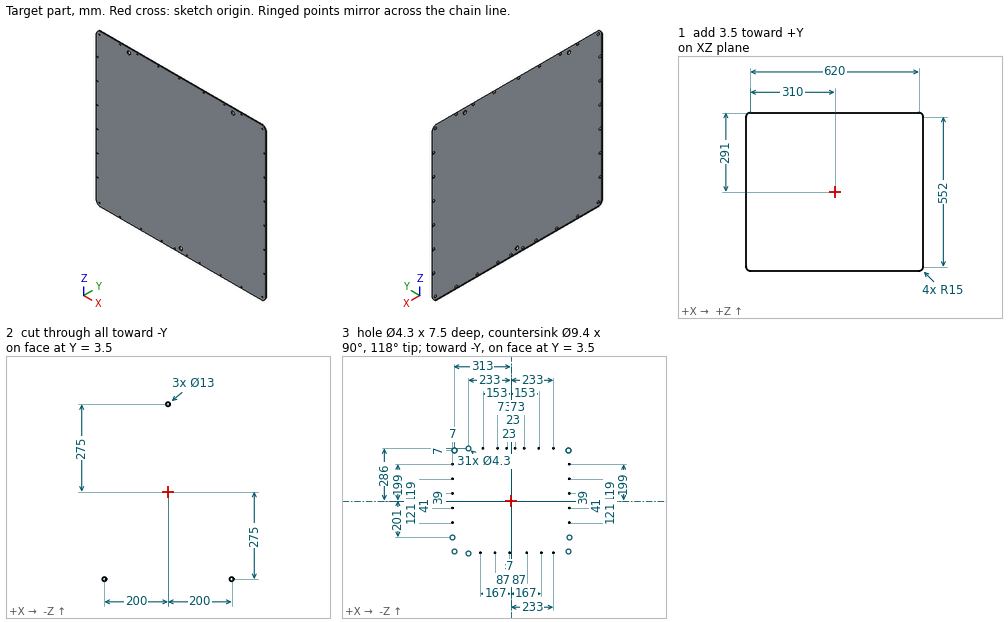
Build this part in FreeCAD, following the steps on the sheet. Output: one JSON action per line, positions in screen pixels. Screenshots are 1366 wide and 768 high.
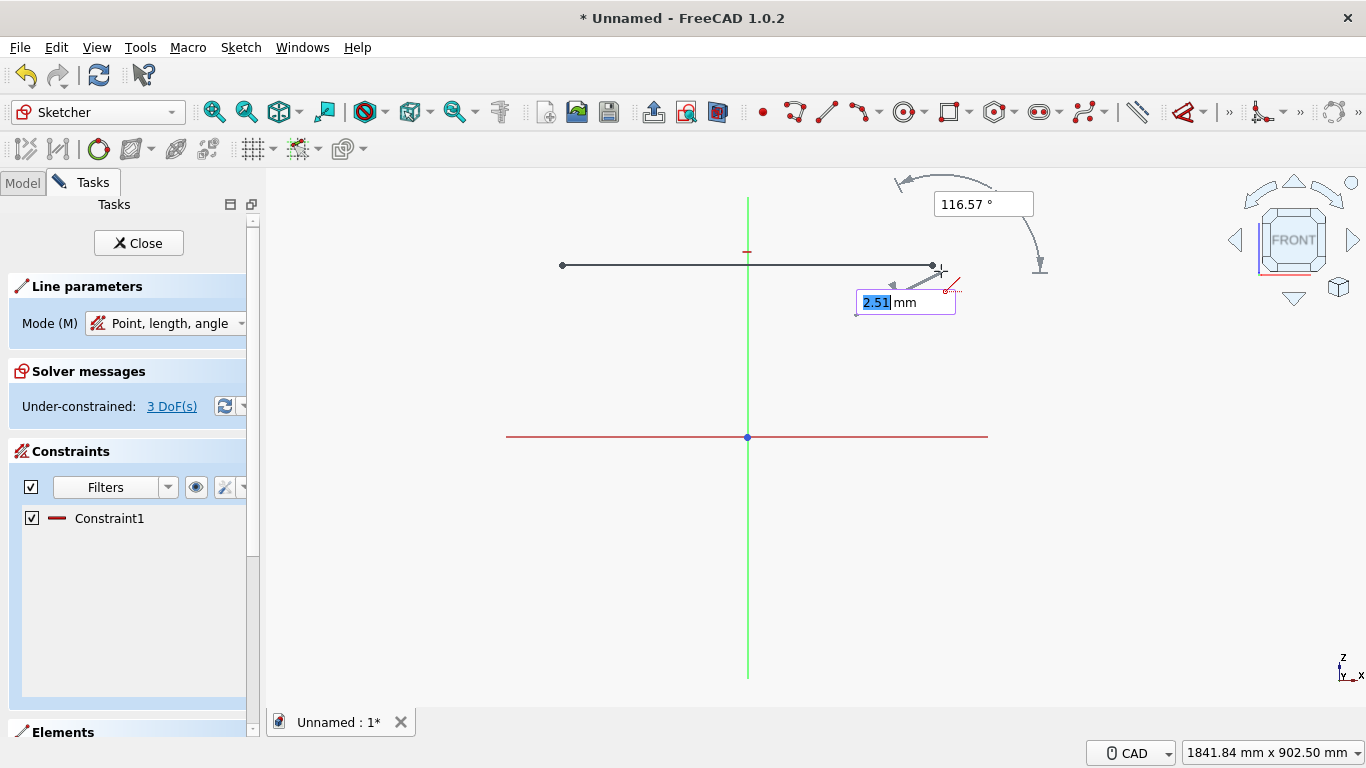
{"action": "left_click", "coordinate": [942, 602]}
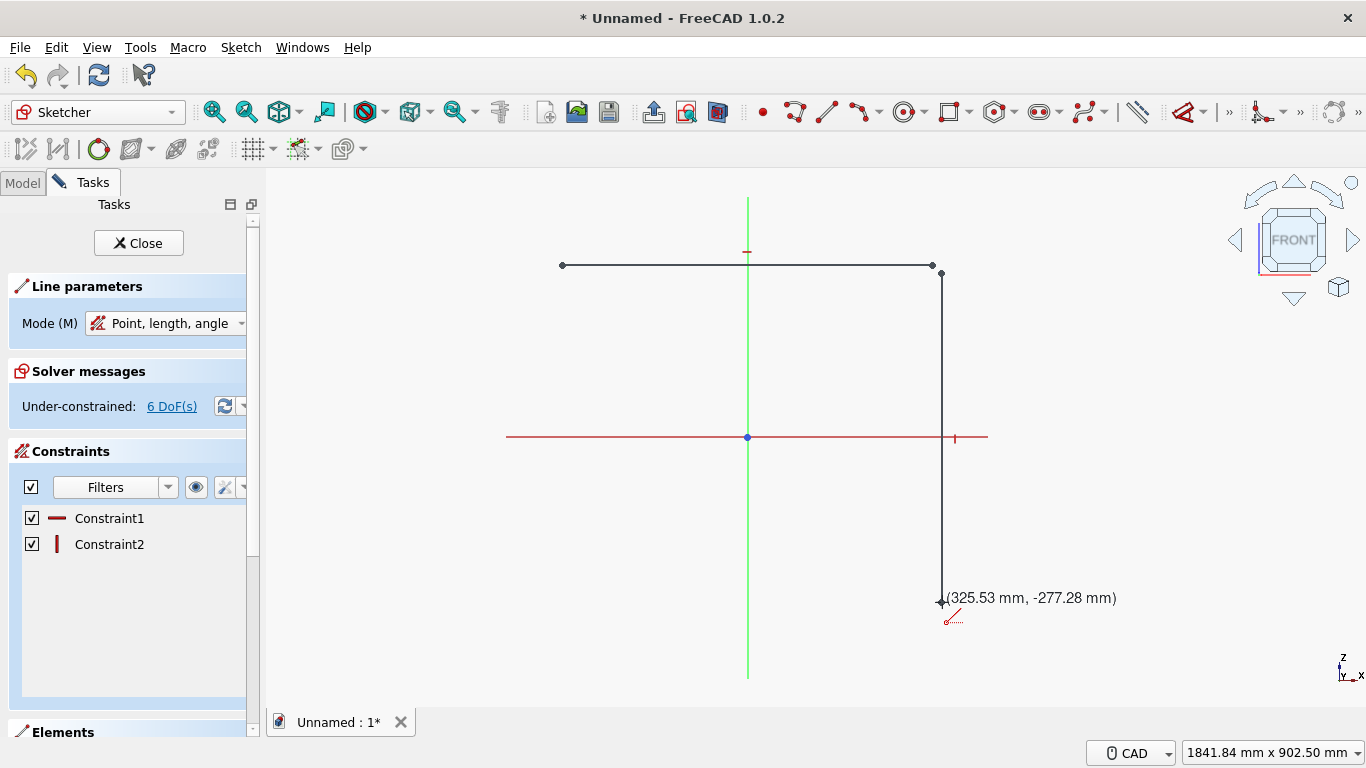
{"action": "scroll", "coordinate": [933, 611], "scroll_direction": "up", "scroll_amount": 2}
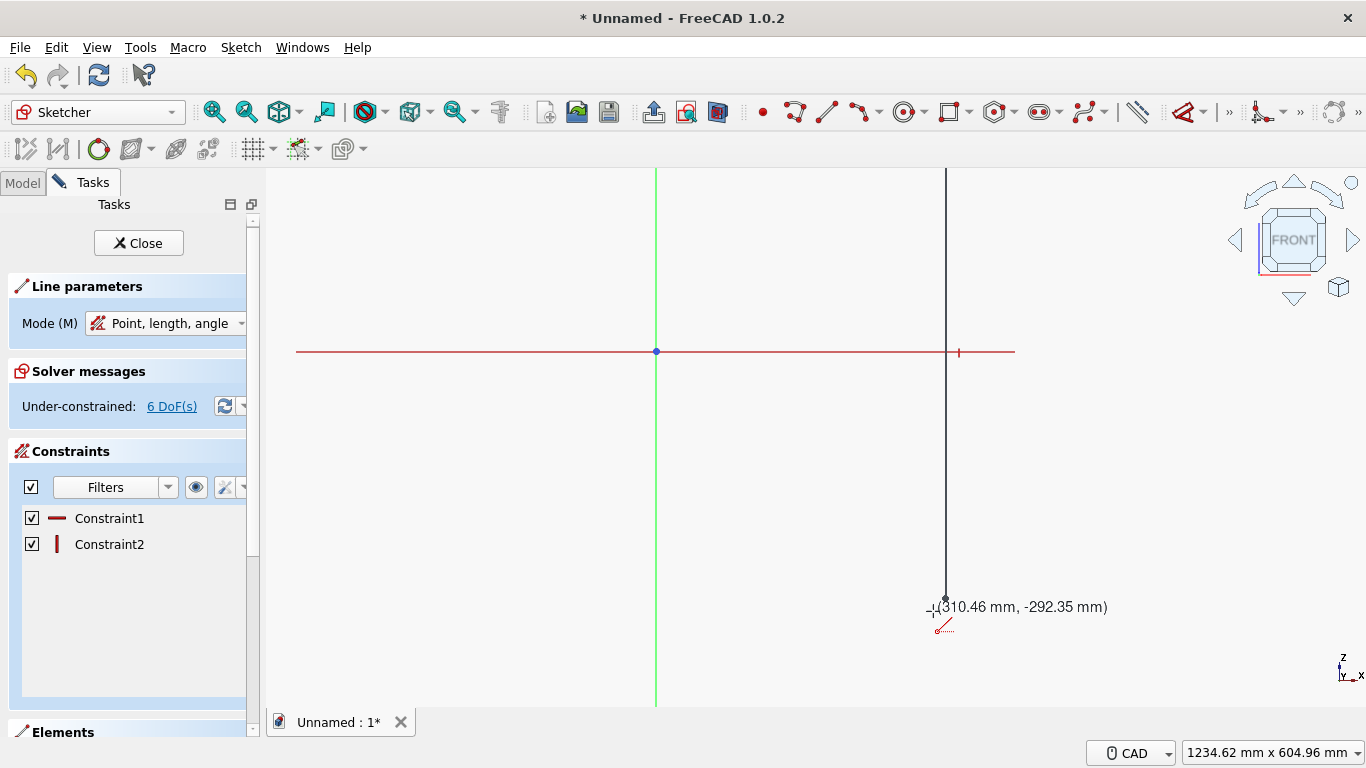
{"action": "left_click", "coordinate": [932, 611]}
{"action": "left_click", "coordinate": [380, 611]}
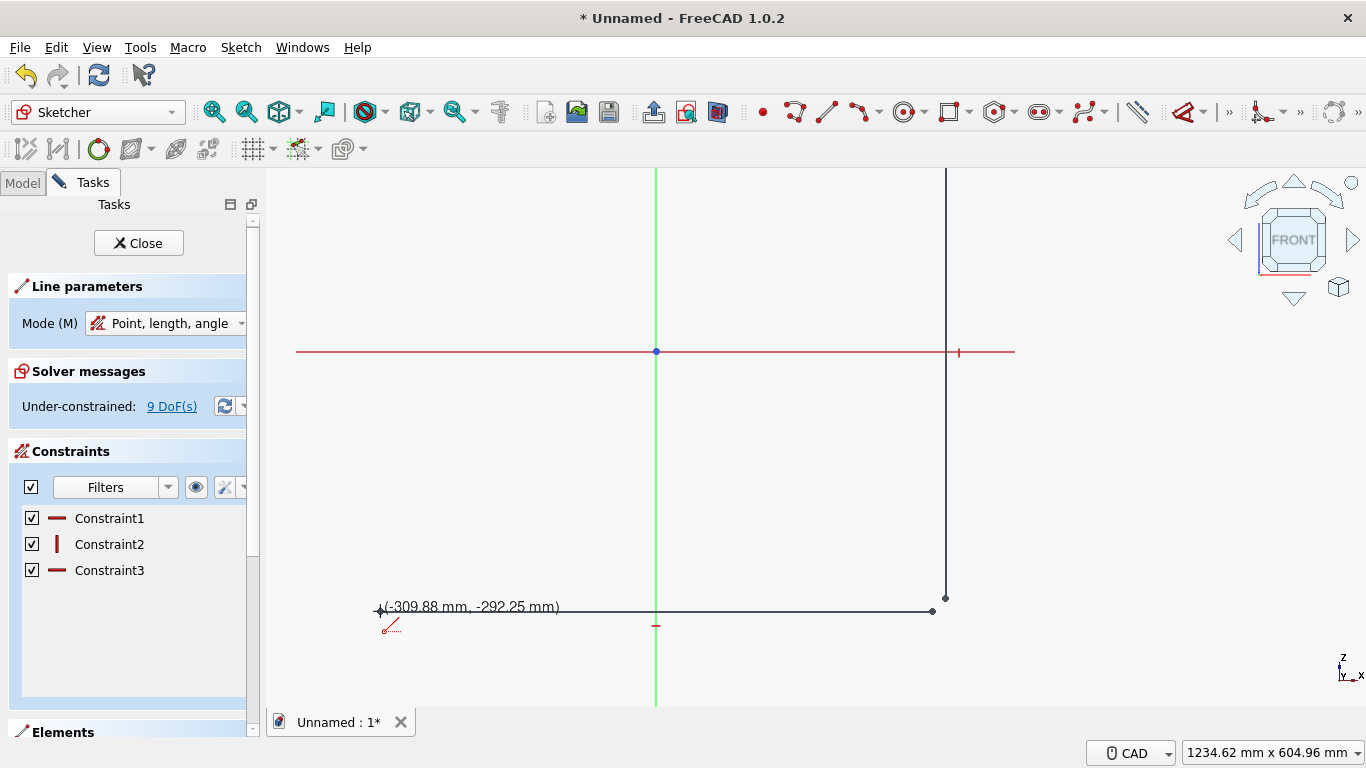
{"action": "left_click", "coordinate": [367, 598]}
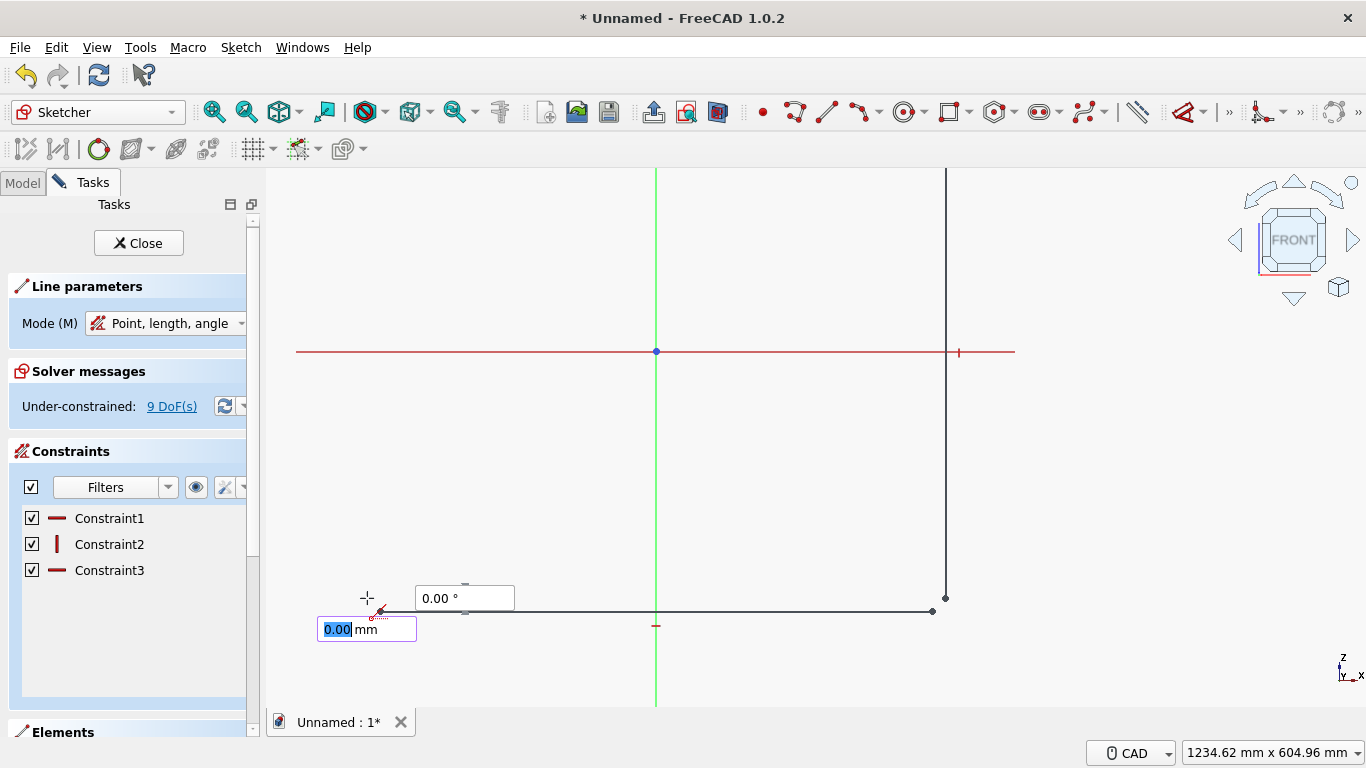
{"action": "scroll", "coordinate": [933, 612], "scroll_direction": "down", "scroll_amount": 2}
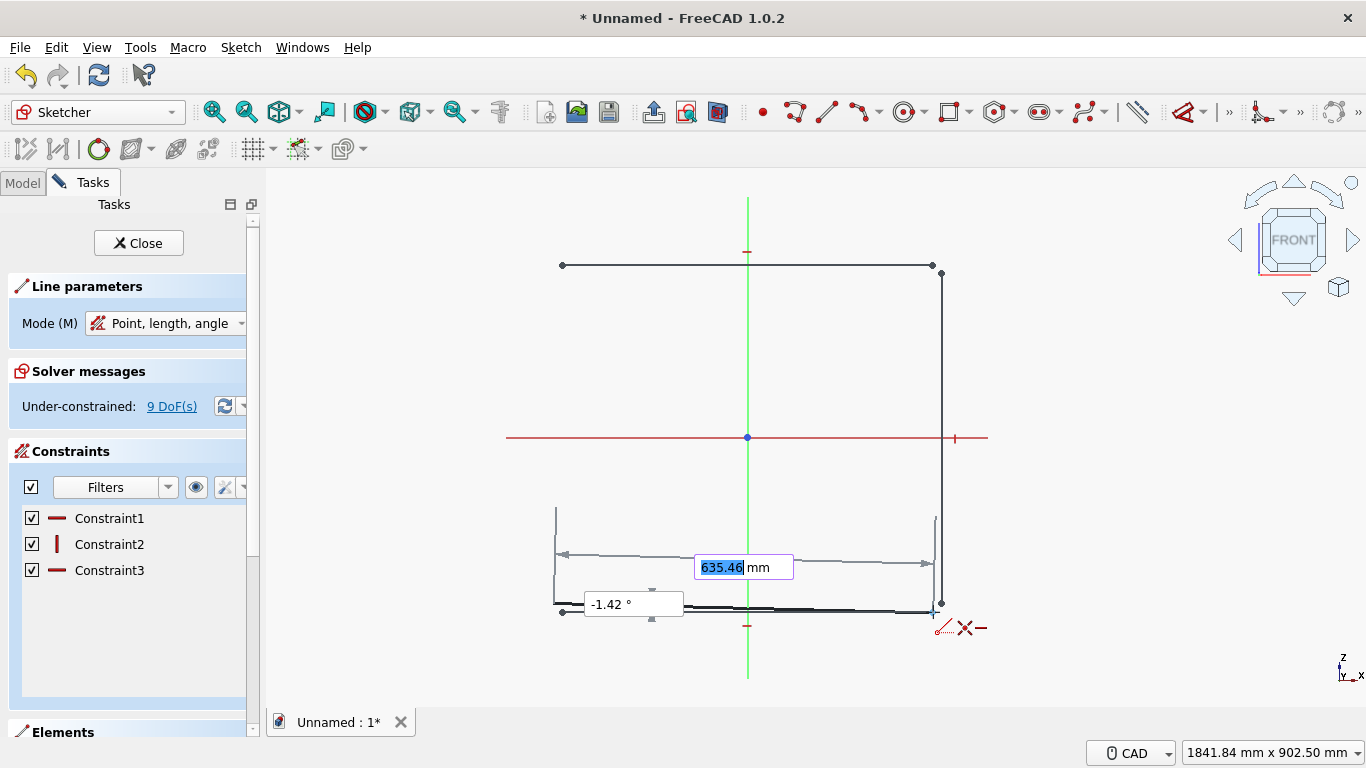
{"action": "scroll", "coordinate": [553, 273], "scroll_direction": "up", "scroll_amount": 2}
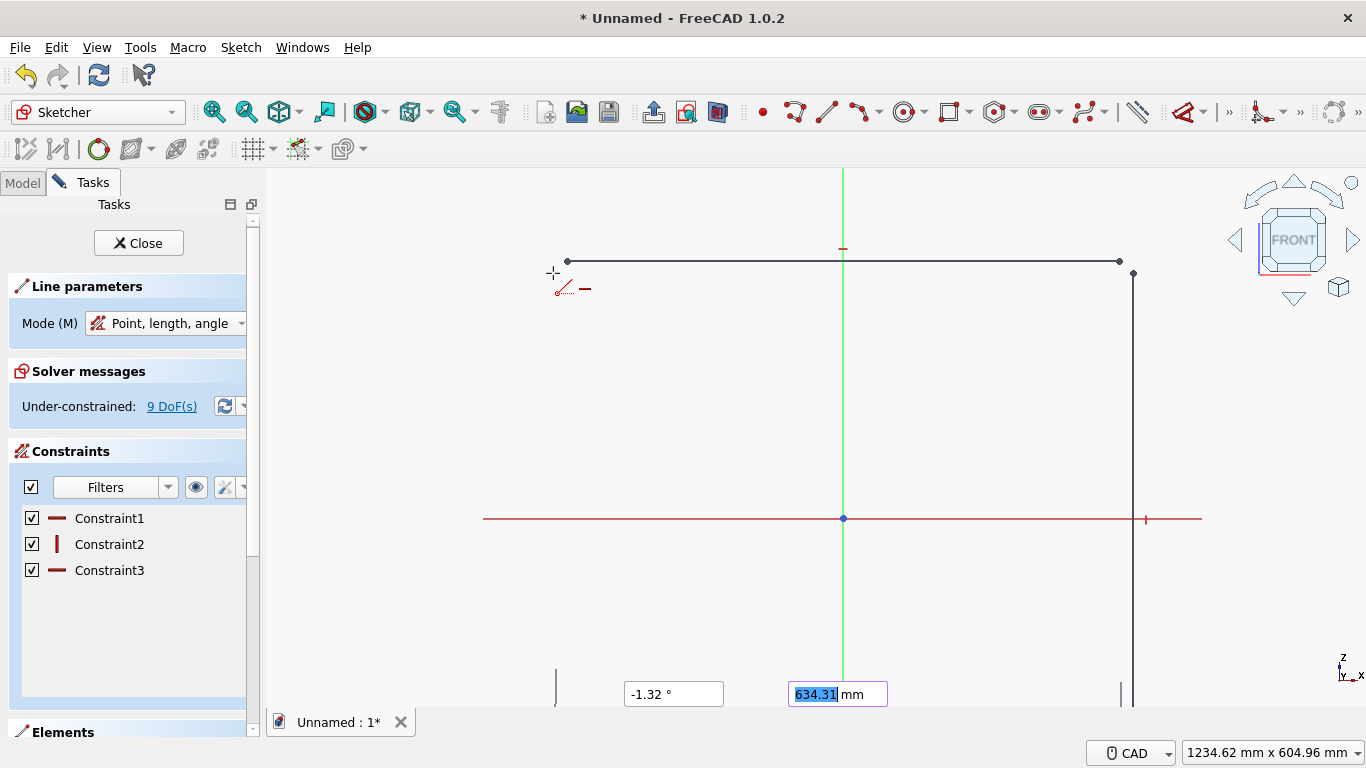
{"action": "left_click", "coordinate": [554, 273]}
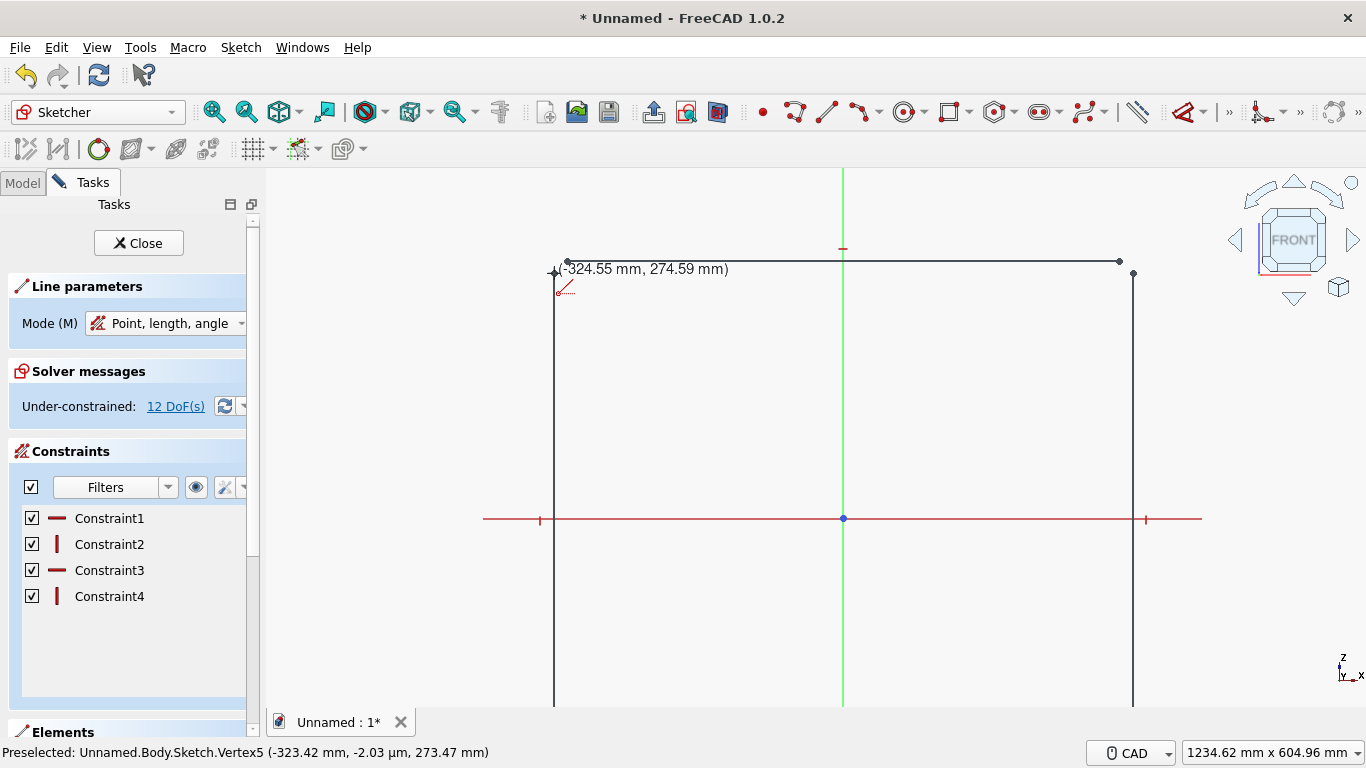
{"action": "left_click", "coordinate": [860, 112]}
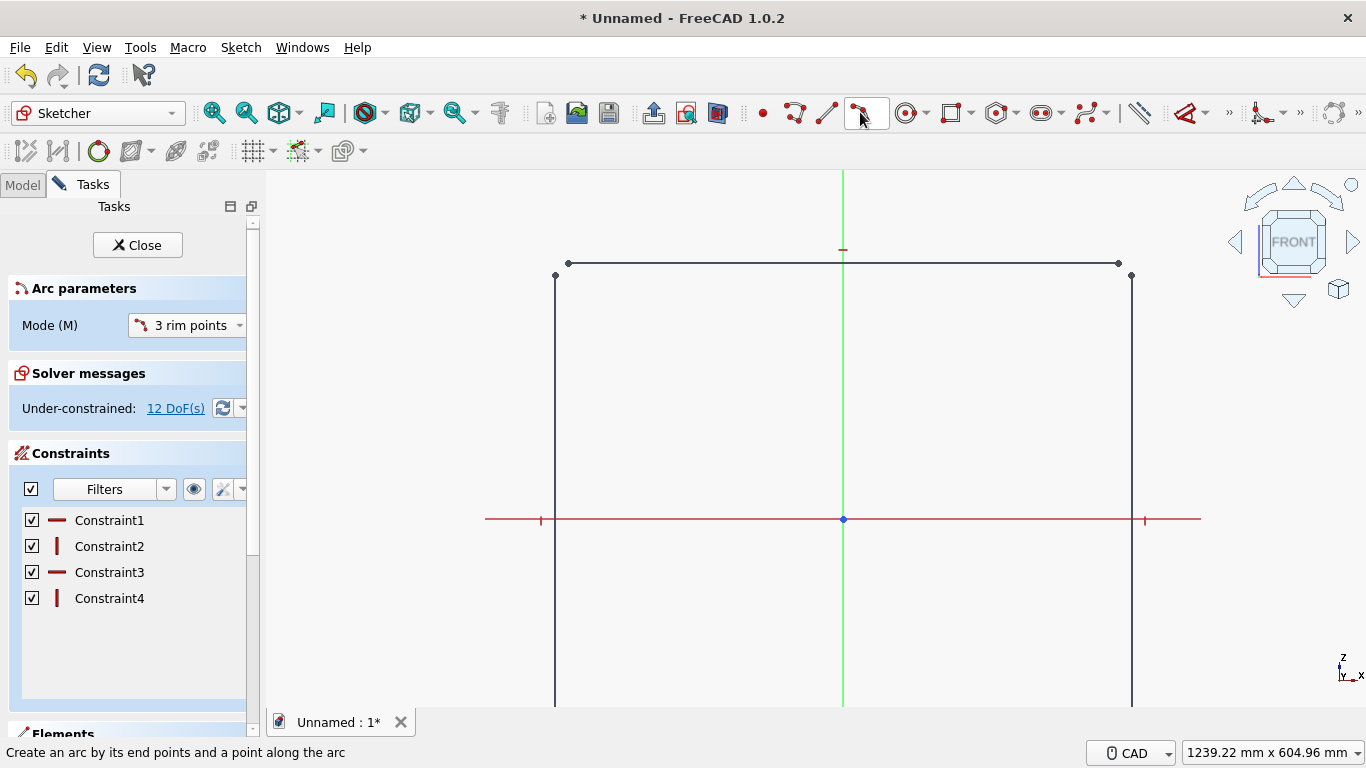
{"action": "left_click", "coordinate": [1118, 263]}
{"action": "left_click", "coordinate": [1132, 275]}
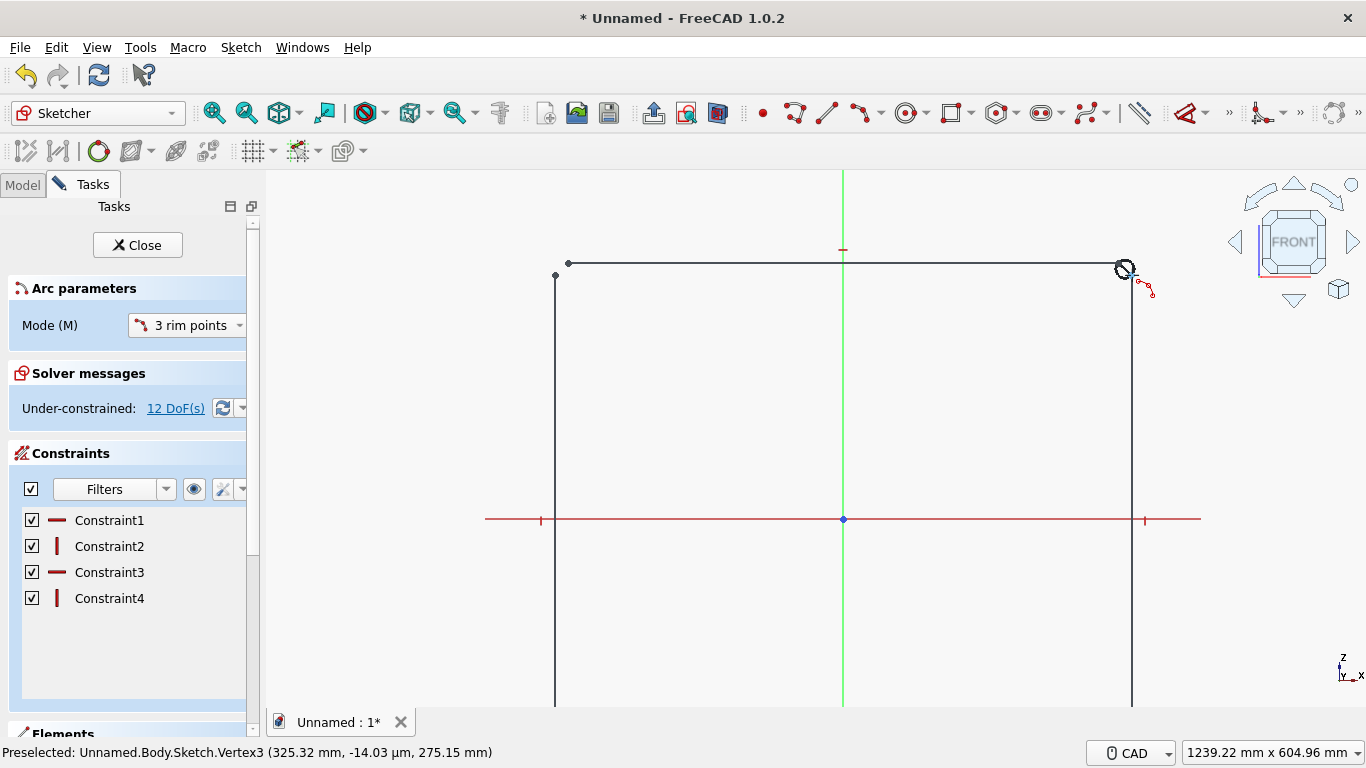
{"action": "scroll", "coordinate": [1128, 265], "scroll_direction": "up", "scroll_amount": 8}